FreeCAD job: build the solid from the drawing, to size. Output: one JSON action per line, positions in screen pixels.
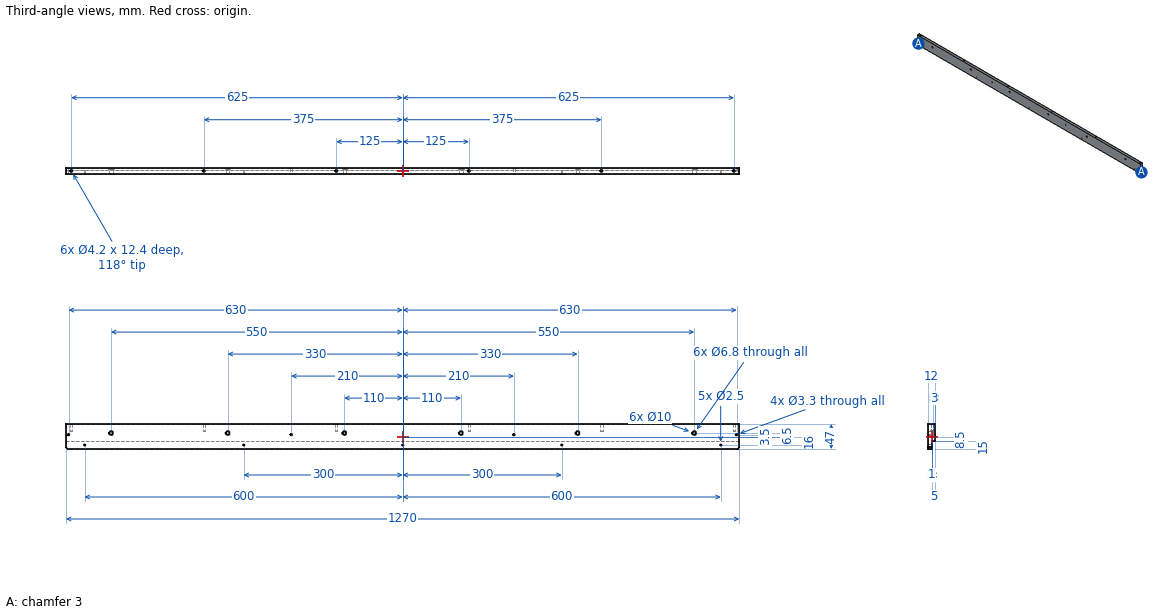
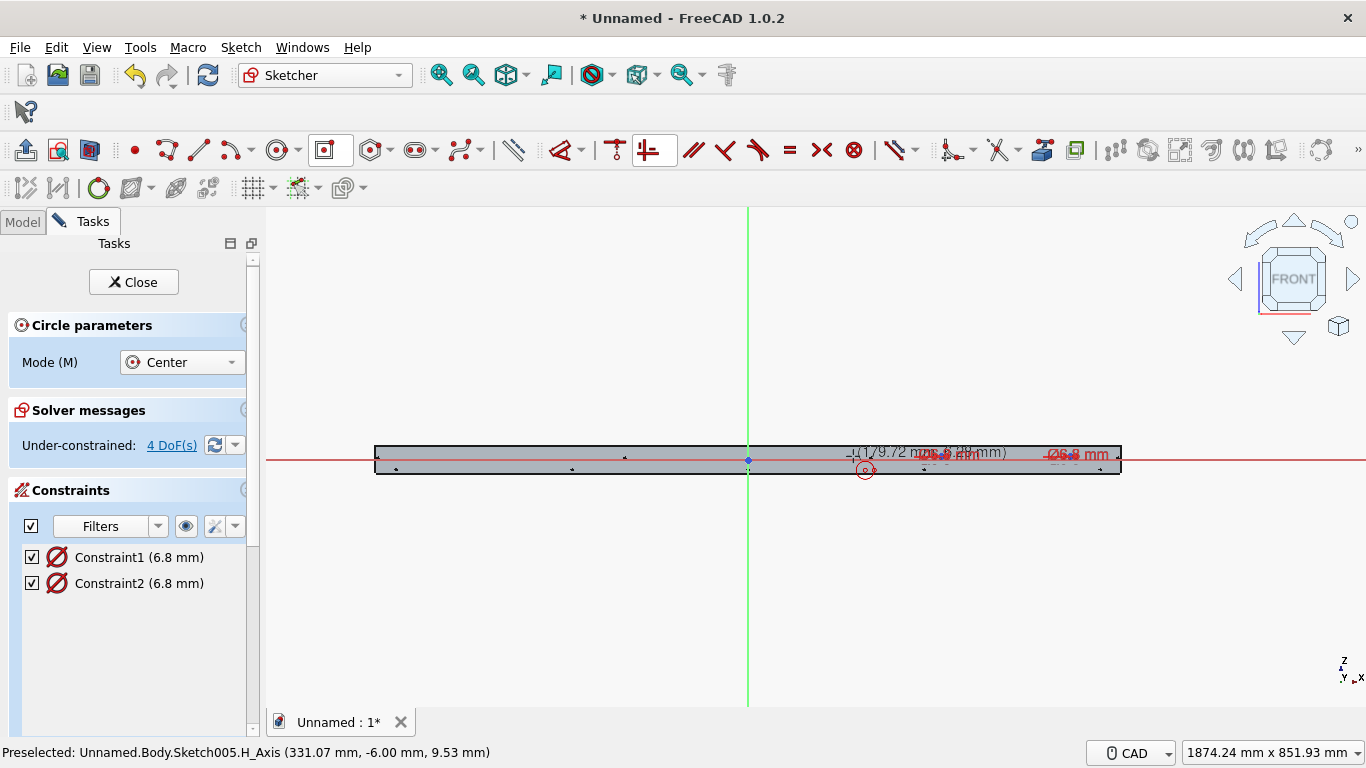
{"action": "scroll", "coordinate": [813, 456], "scroll_direction": "up", "scroll_amount": 8}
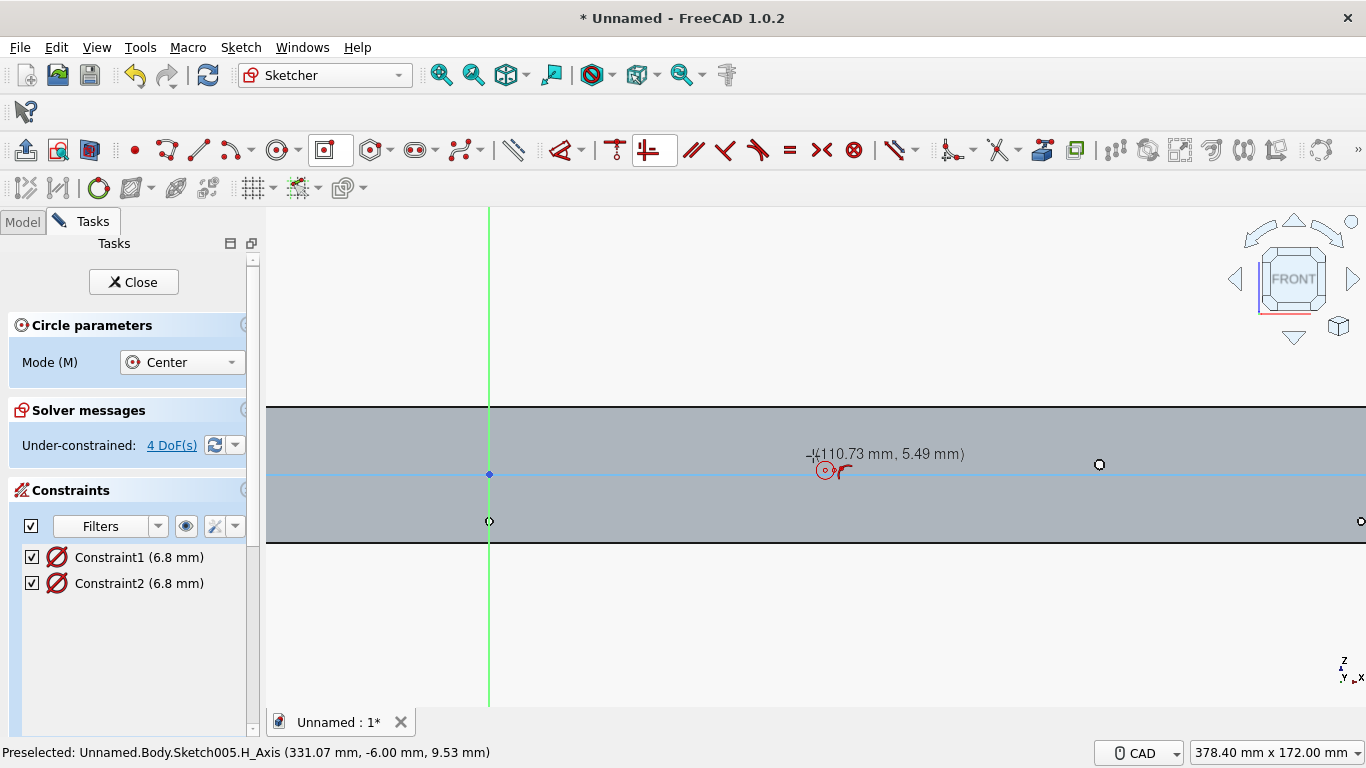
{"action": "left_click", "coordinate": [809, 456]}
{"action": "mouse_move", "coordinate": [816, 449]}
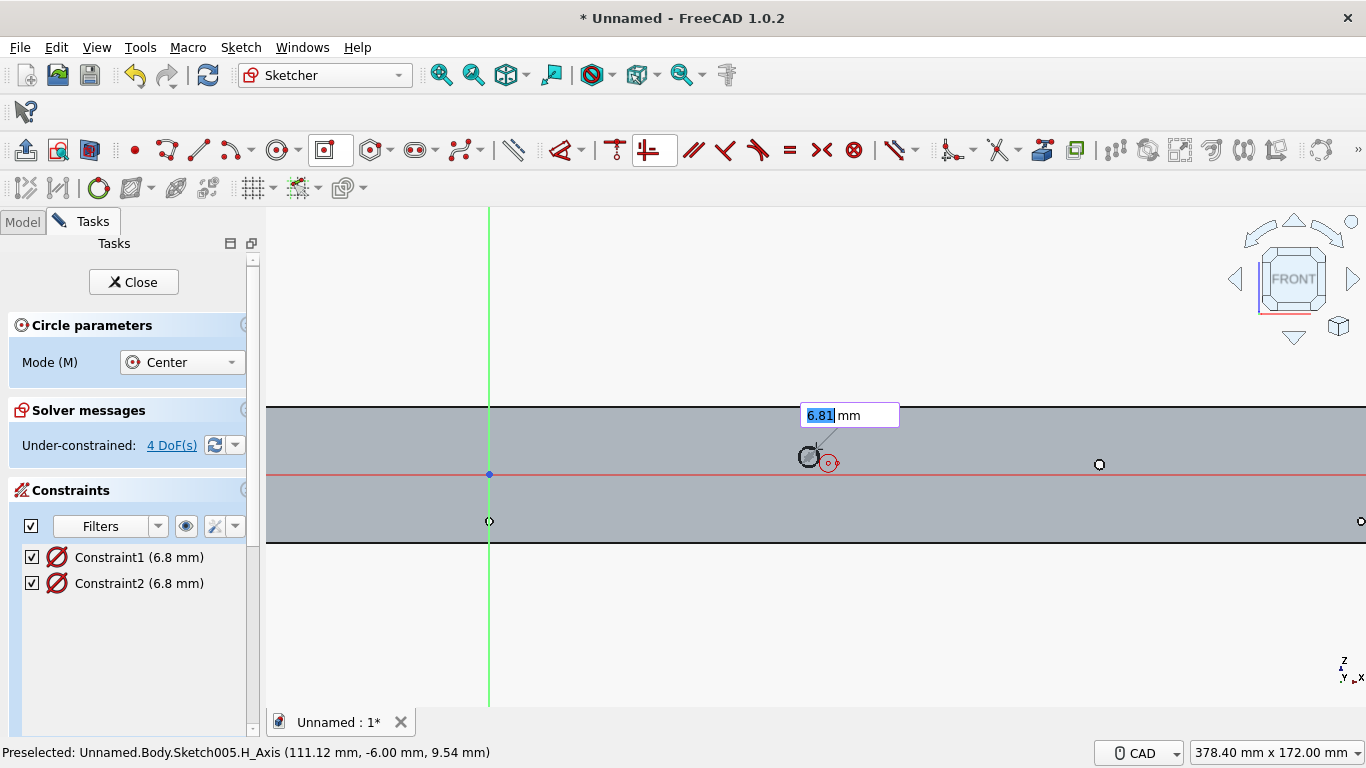
{"action": "type", "text": "6.8"}
{"action": "key", "text": "Return"}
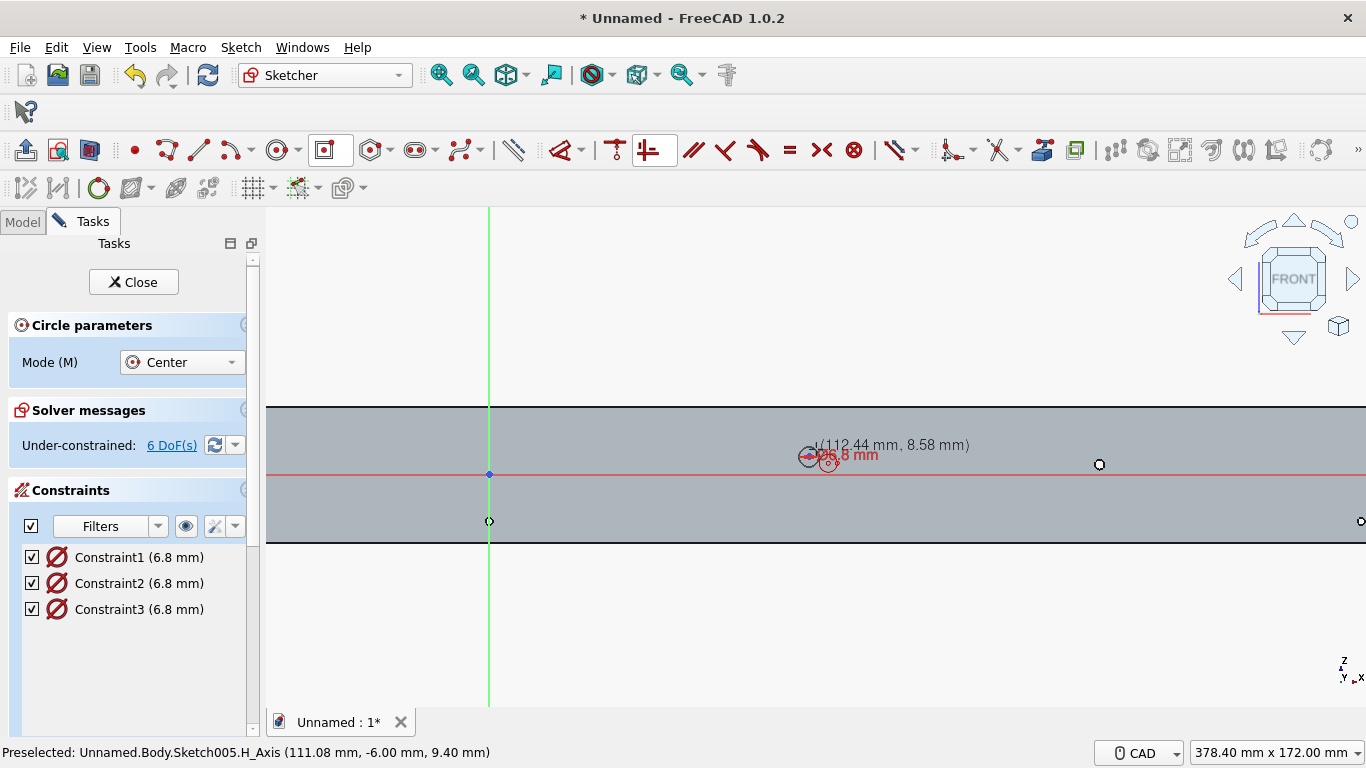
{"action": "scroll", "coordinate": [813, 456], "scroll_direction": "down", "scroll_amount": 8}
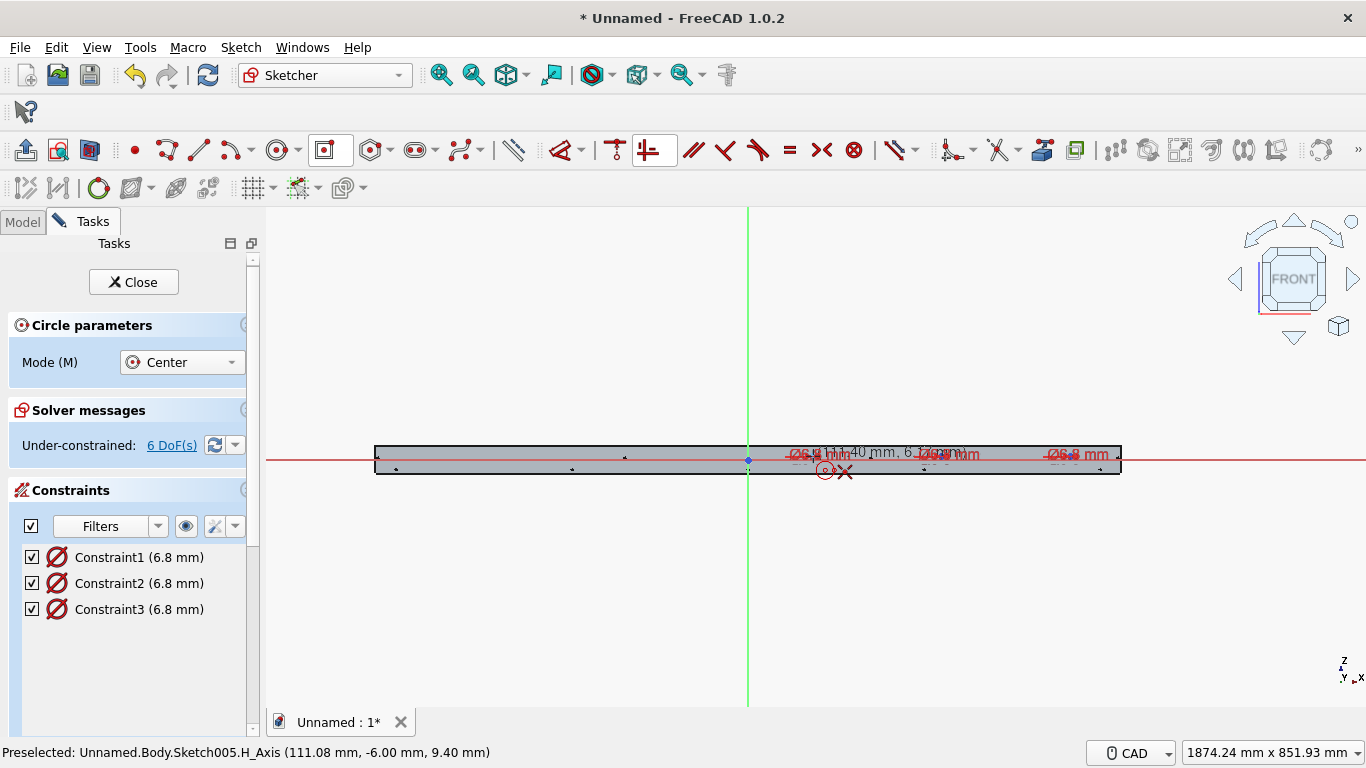
{"action": "scroll", "coordinate": [683, 456], "scroll_direction": "up", "scroll_amount": 13}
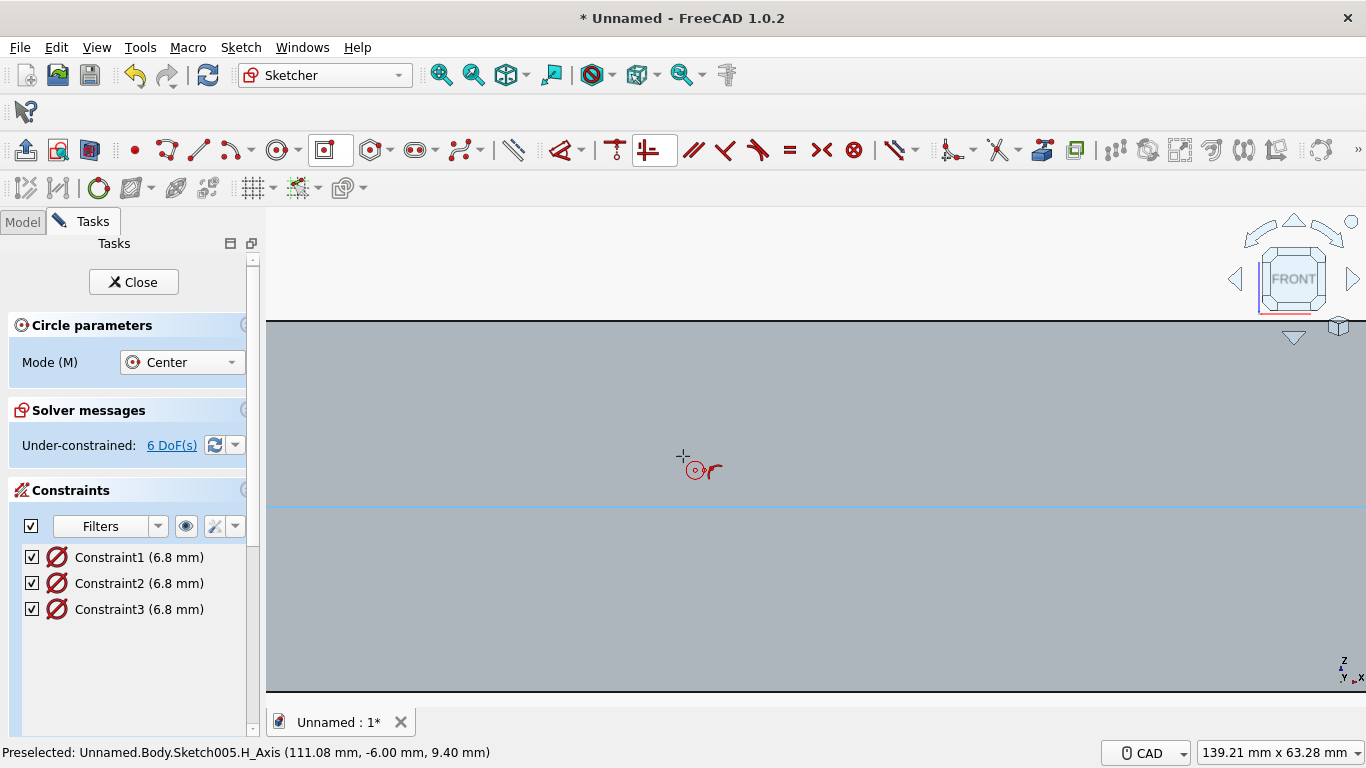
{"action": "scroll", "coordinate": [683, 456], "scroll_direction": "down", "scroll_amount": 13}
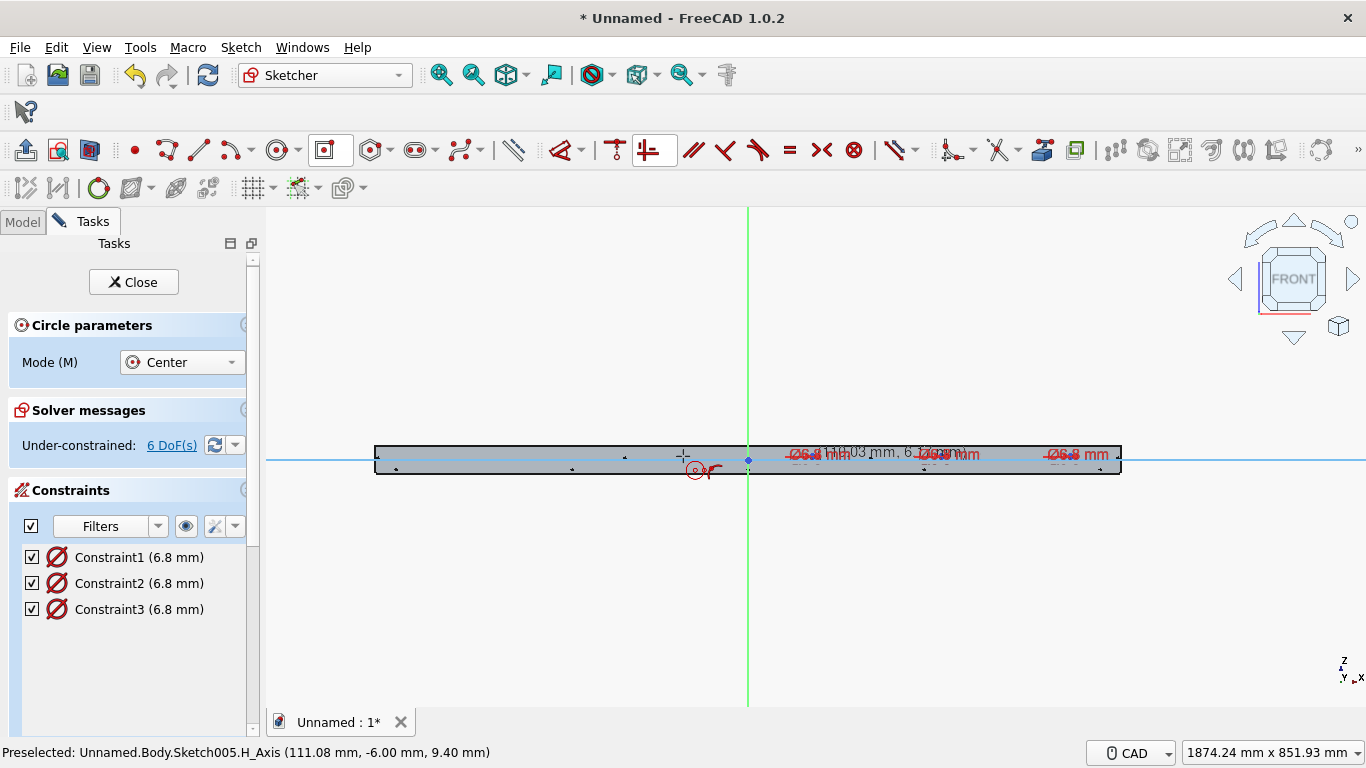
{"action": "scroll", "coordinate": [683, 456], "scroll_direction": "up", "scroll_amount": 8}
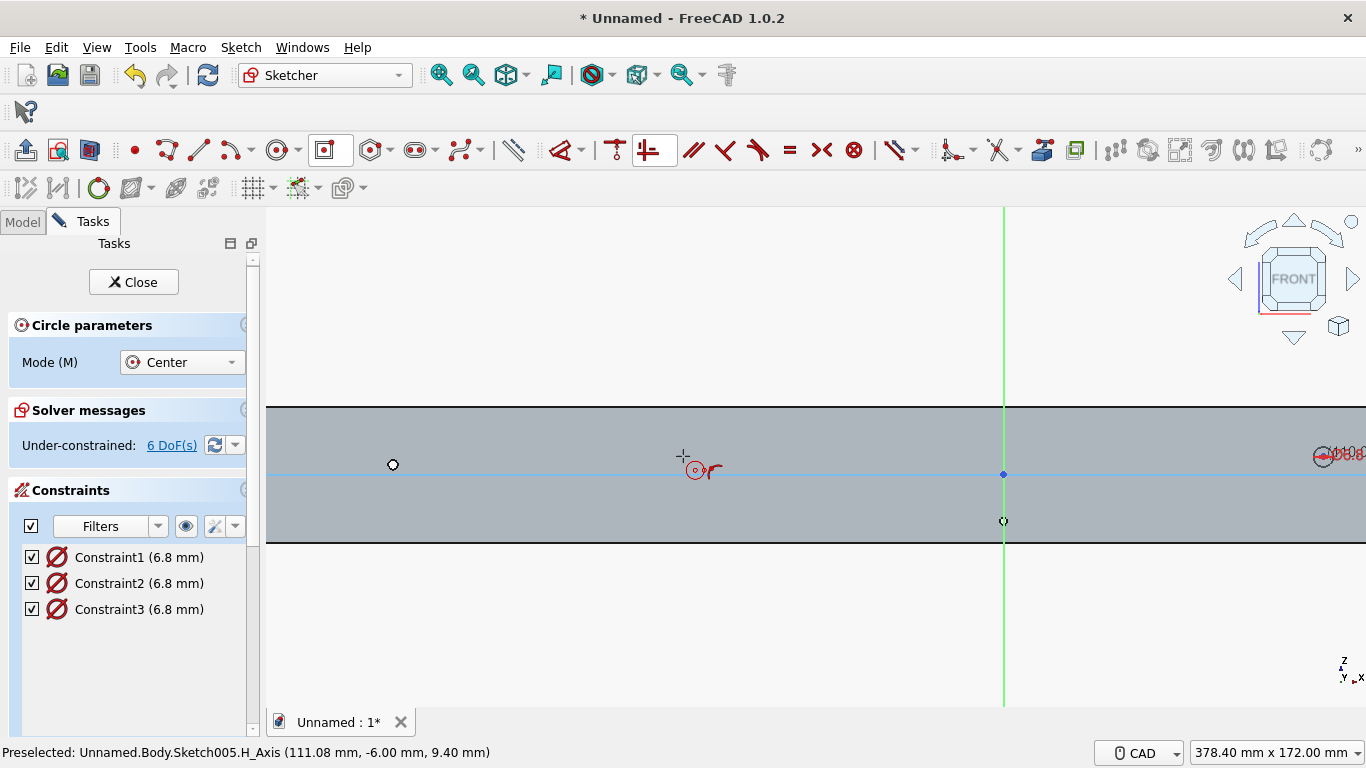
{"action": "left_click", "coordinate": [684, 456]}
{"action": "mouse_move", "coordinate": [691, 449]}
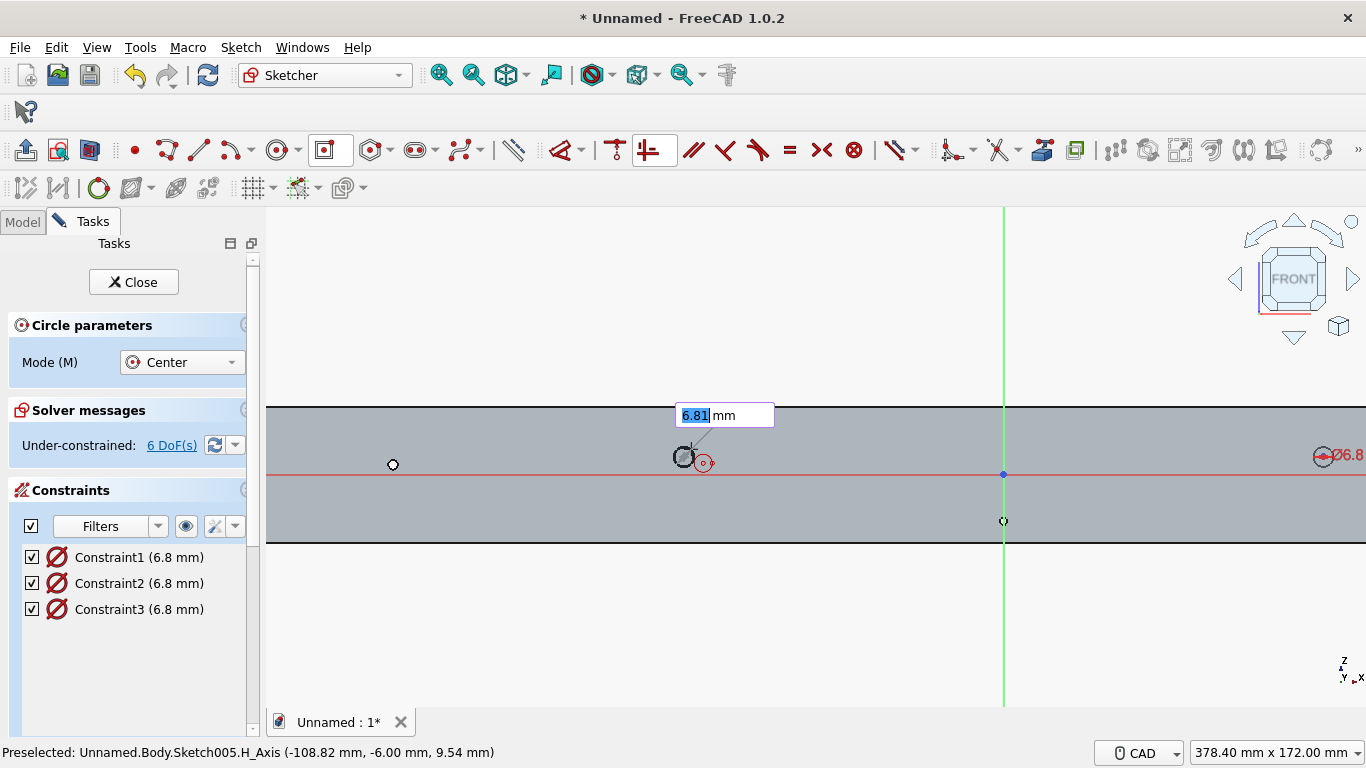
{"action": "type", "text": "6.8"}
{"action": "key", "text": "Return"}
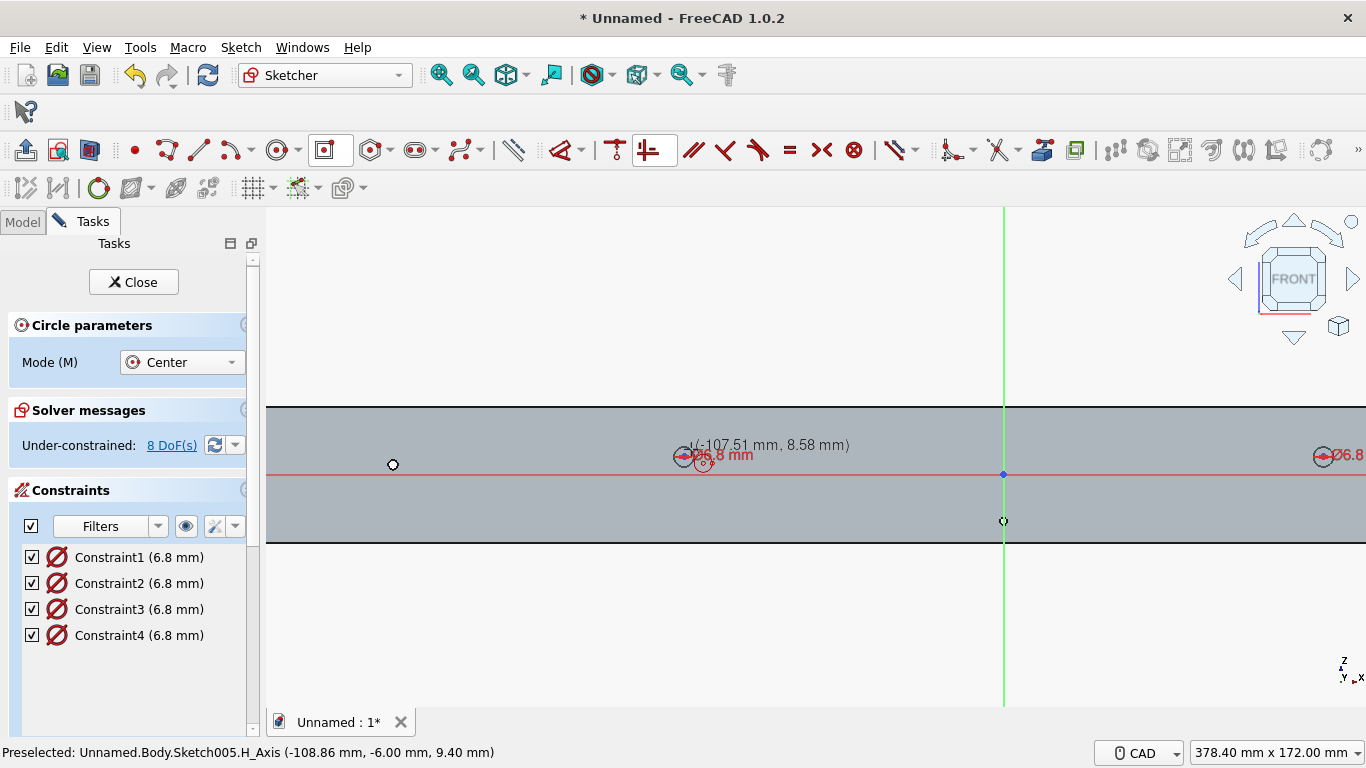
{"action": "scroll", "coordinate": [683, 456], "scroll_direction": "down", "scroll_amount": 8}